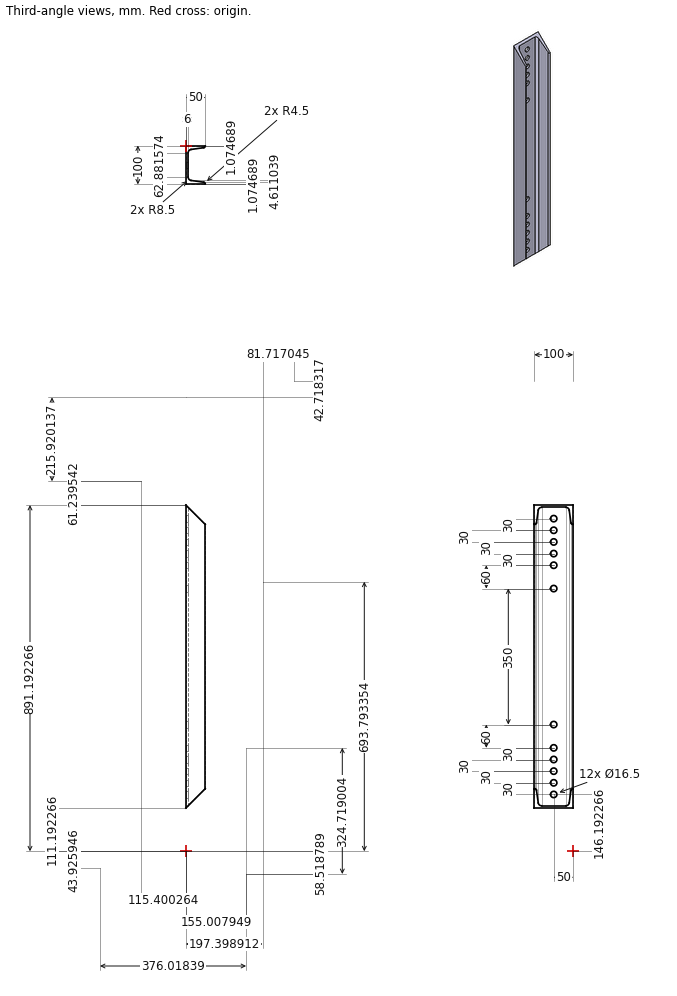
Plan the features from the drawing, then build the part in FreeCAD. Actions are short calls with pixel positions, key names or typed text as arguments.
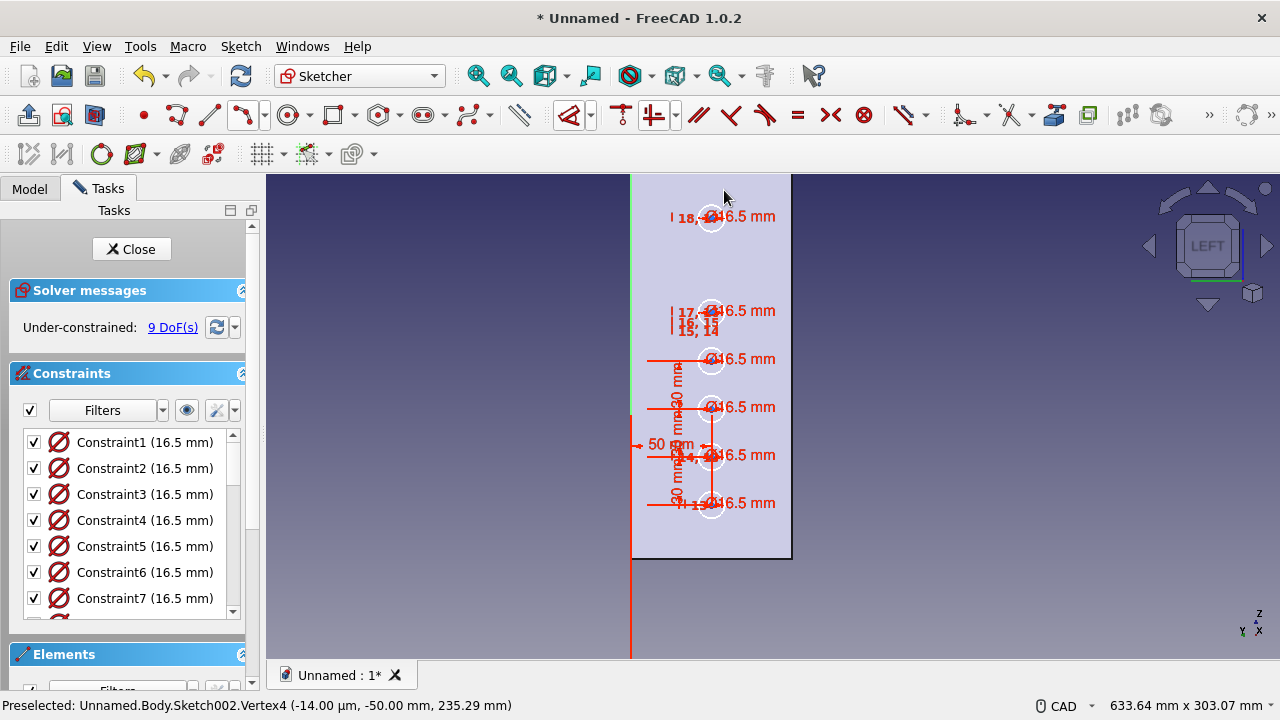
click(712, 361)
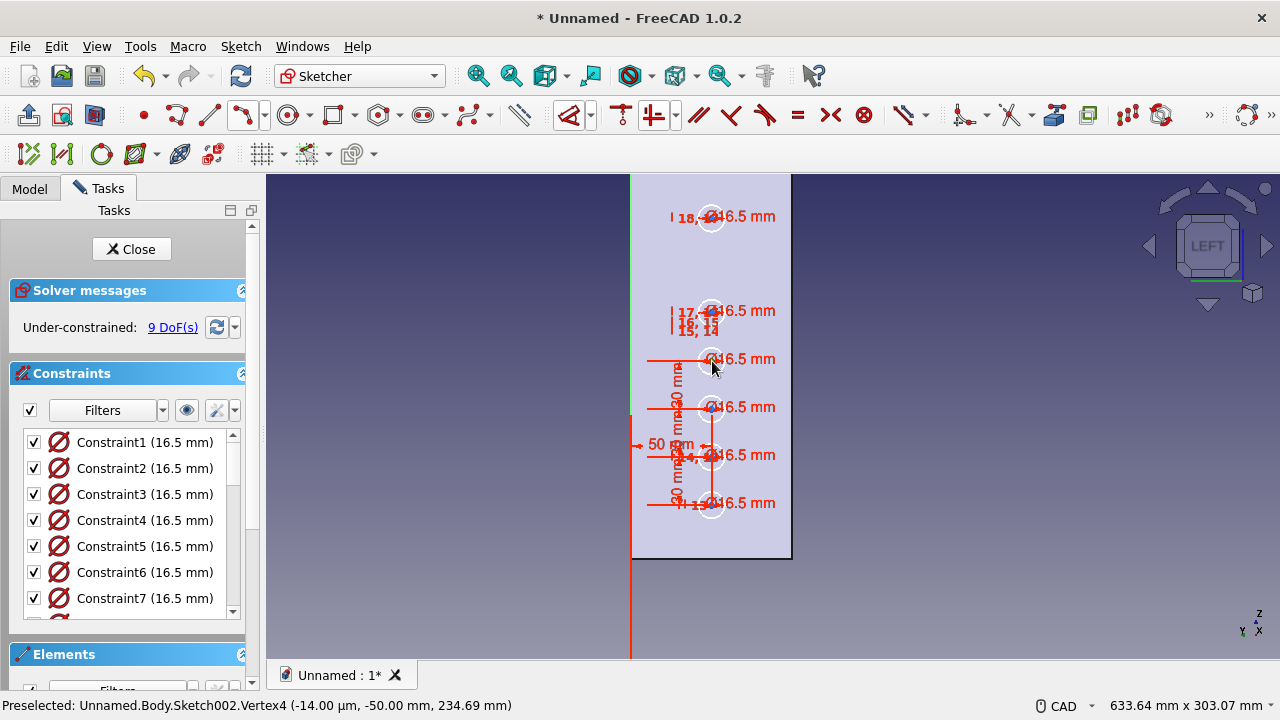
click(712, 313)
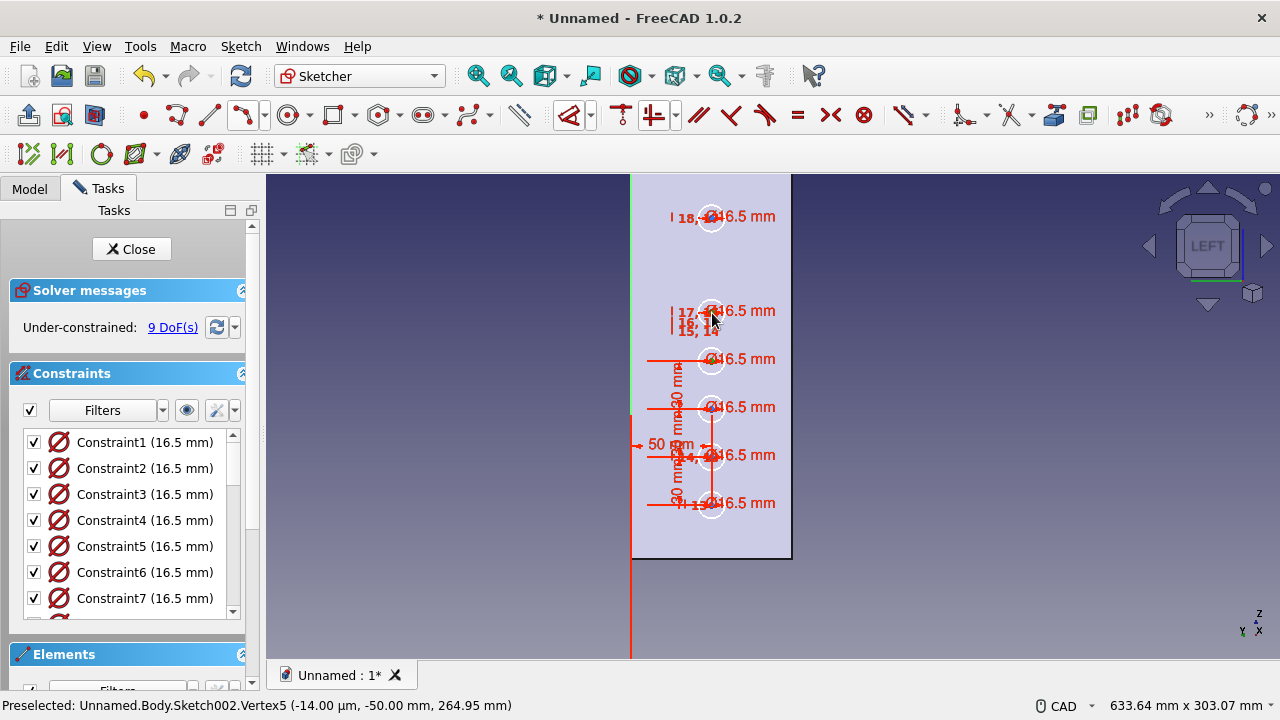
key(i)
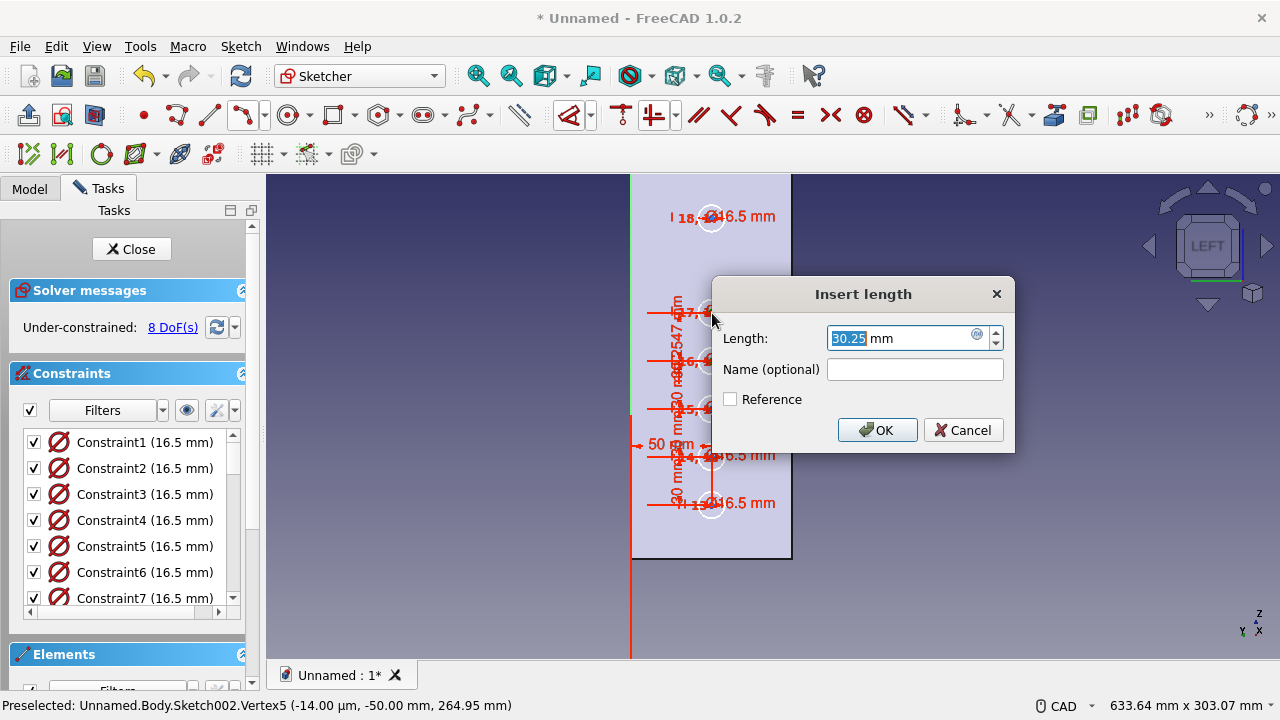
text(30)
key(Return)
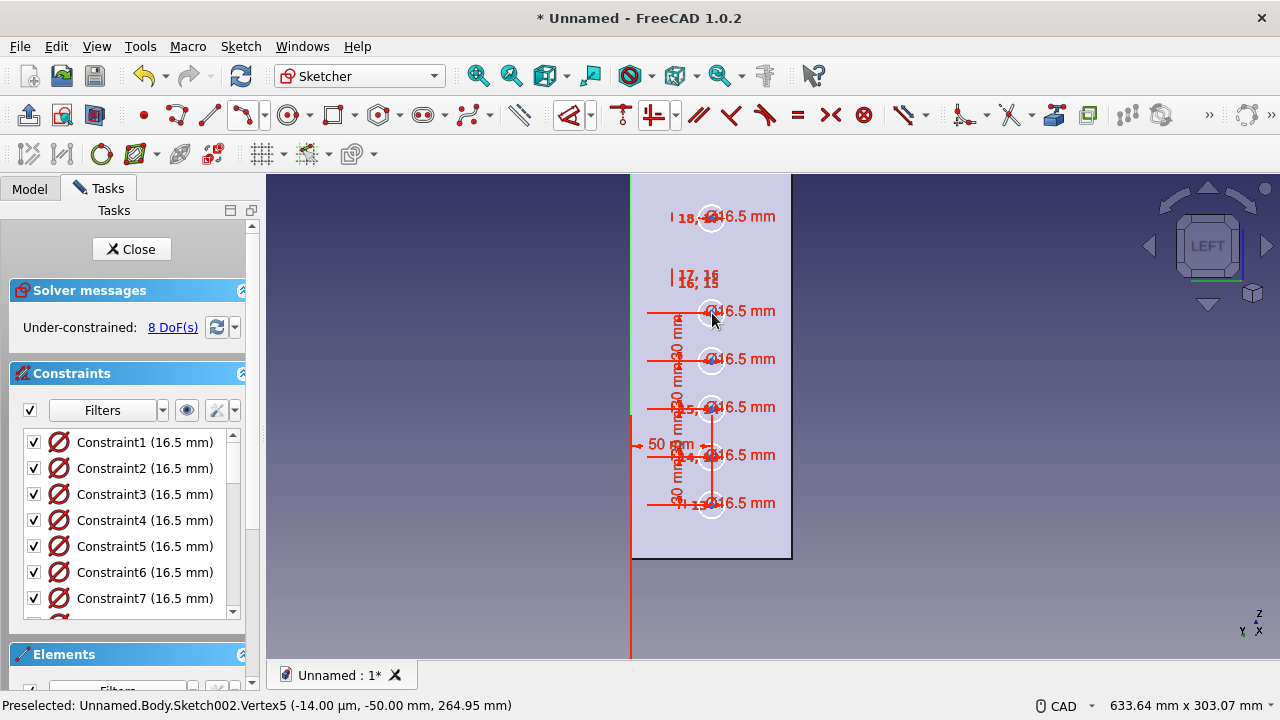
click(712, 313)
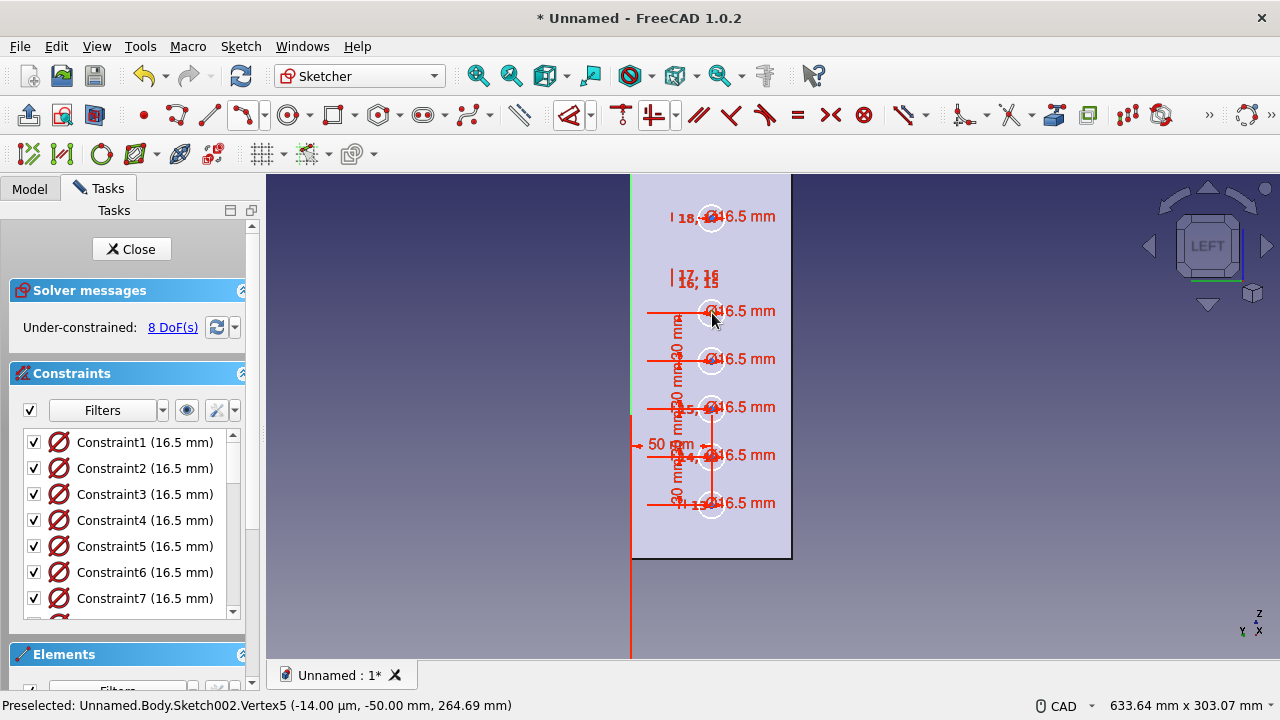
click(712, 218)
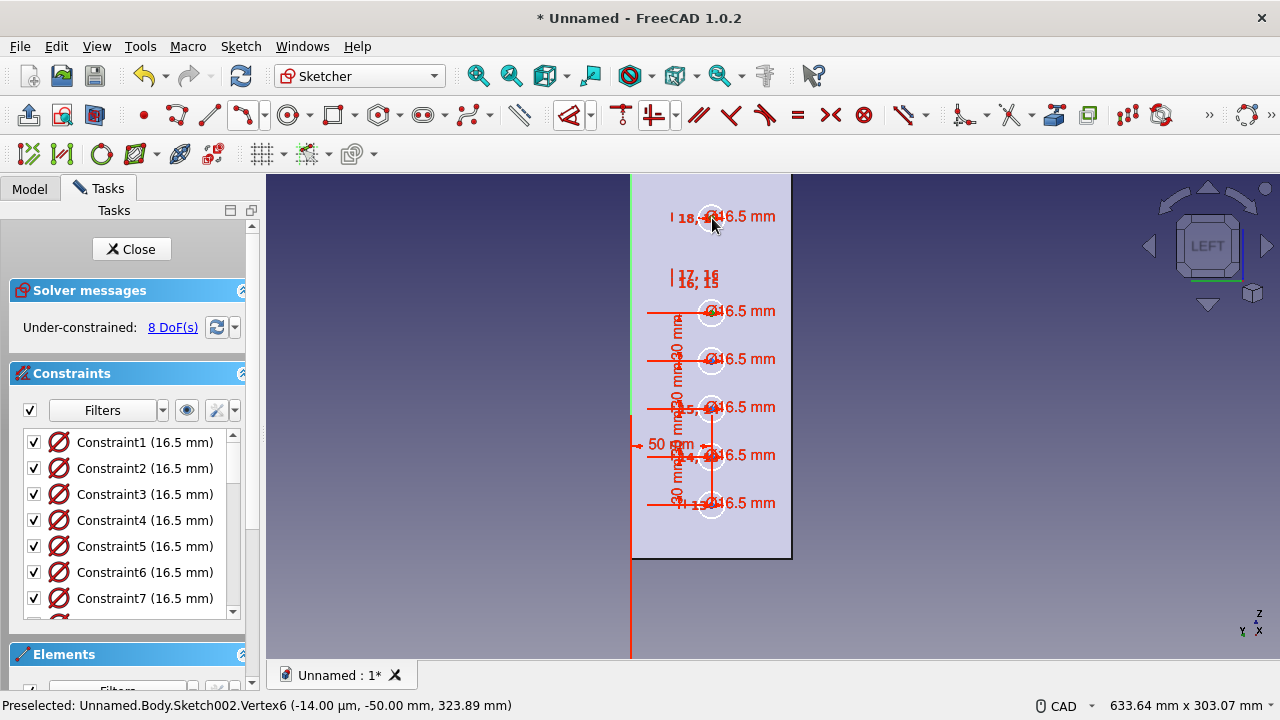
click(590, 116)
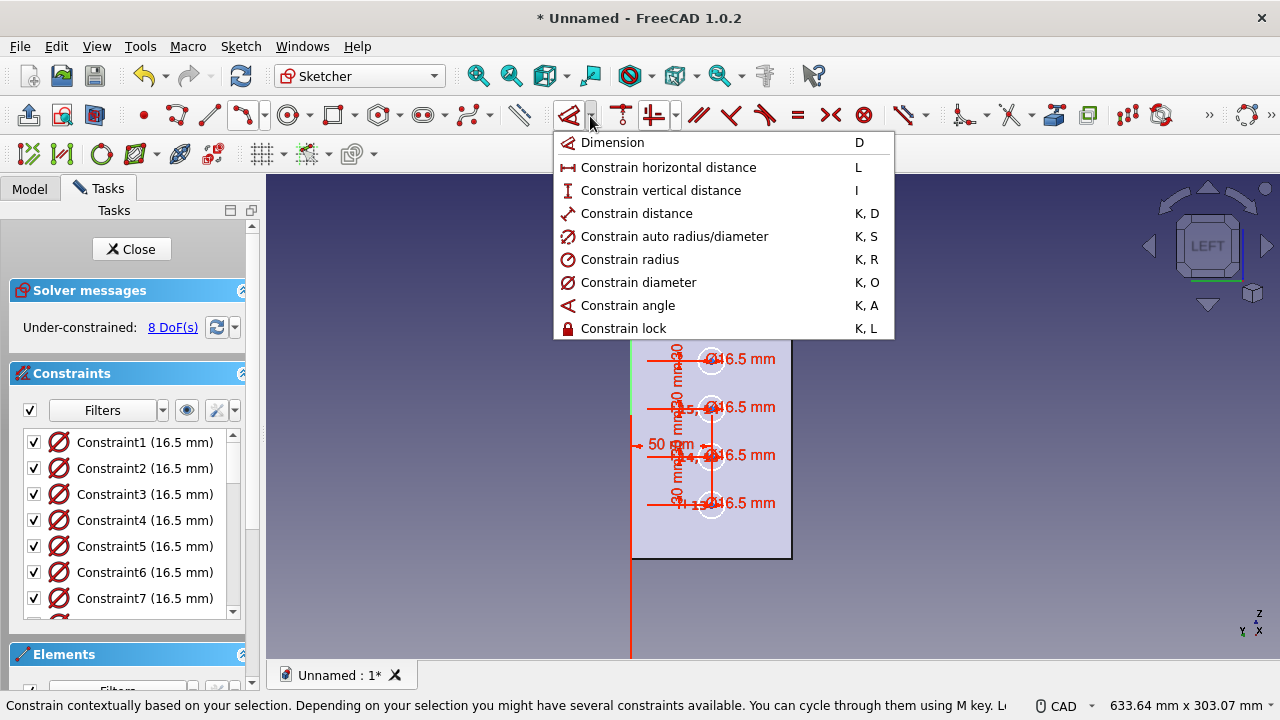
click(724, 190)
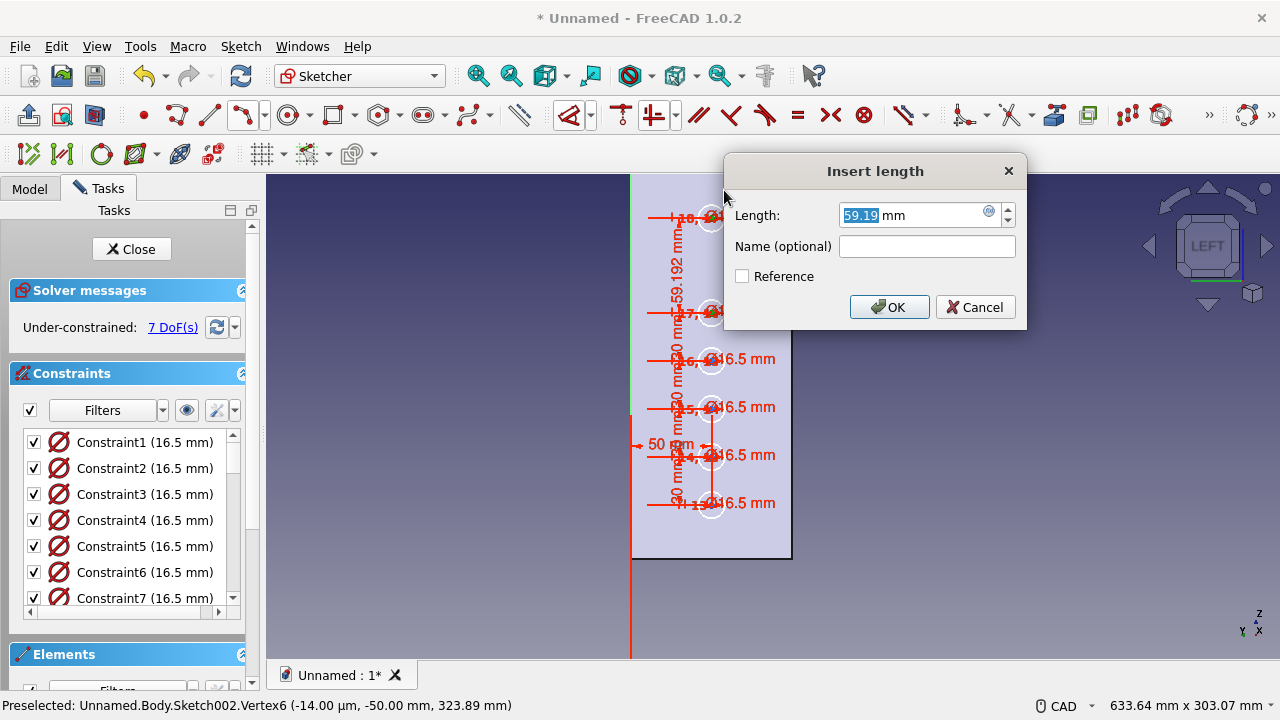
text(60)
key(Return)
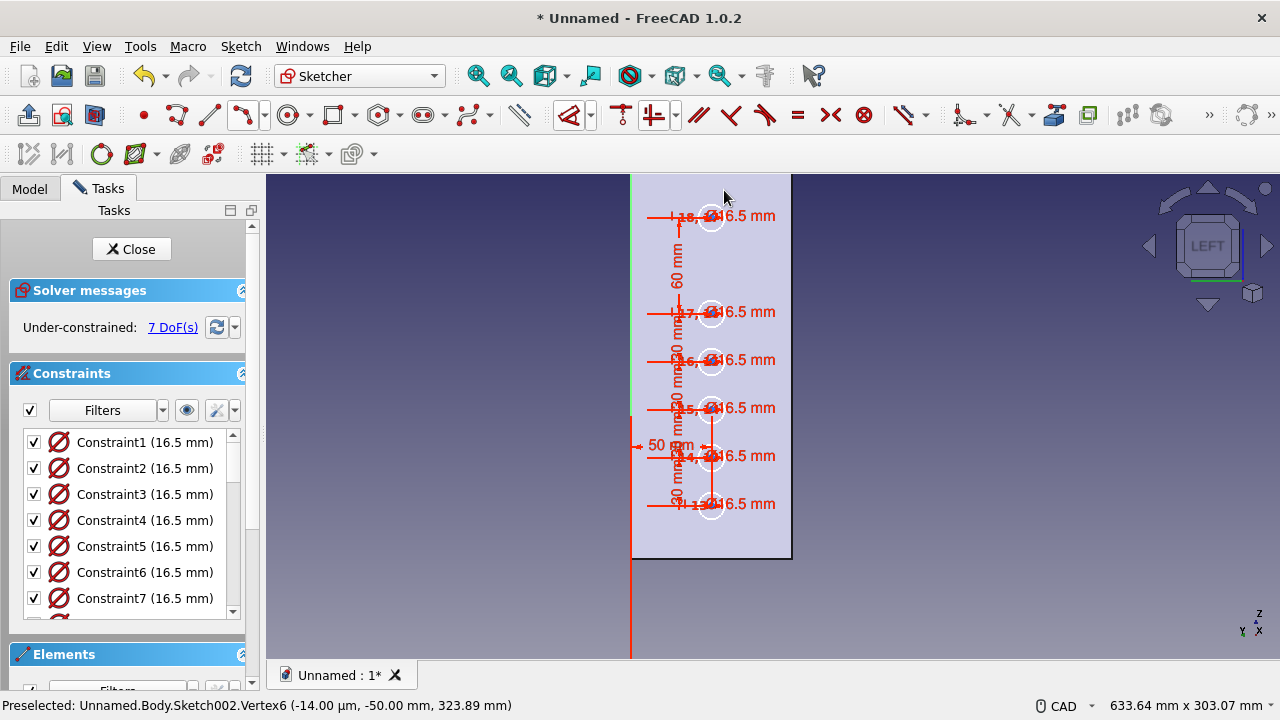
scroll(711, 510, down, 8)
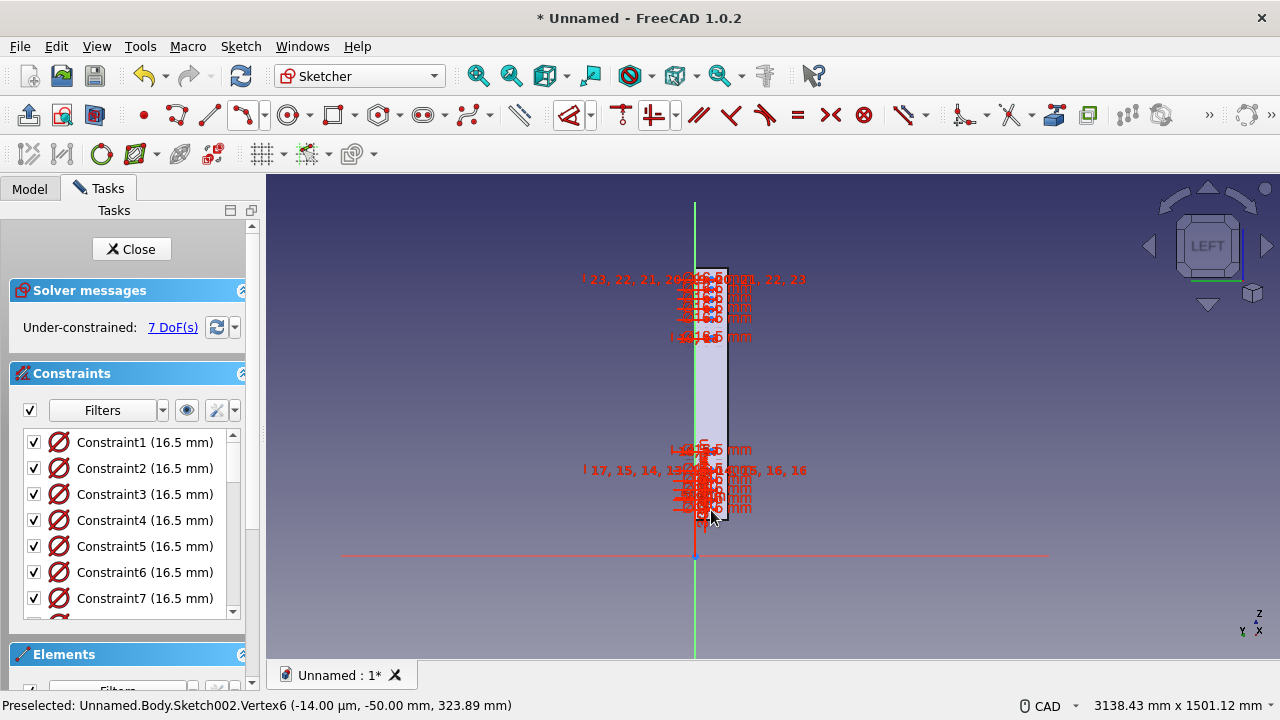
scroll(711, 339, up, 4)